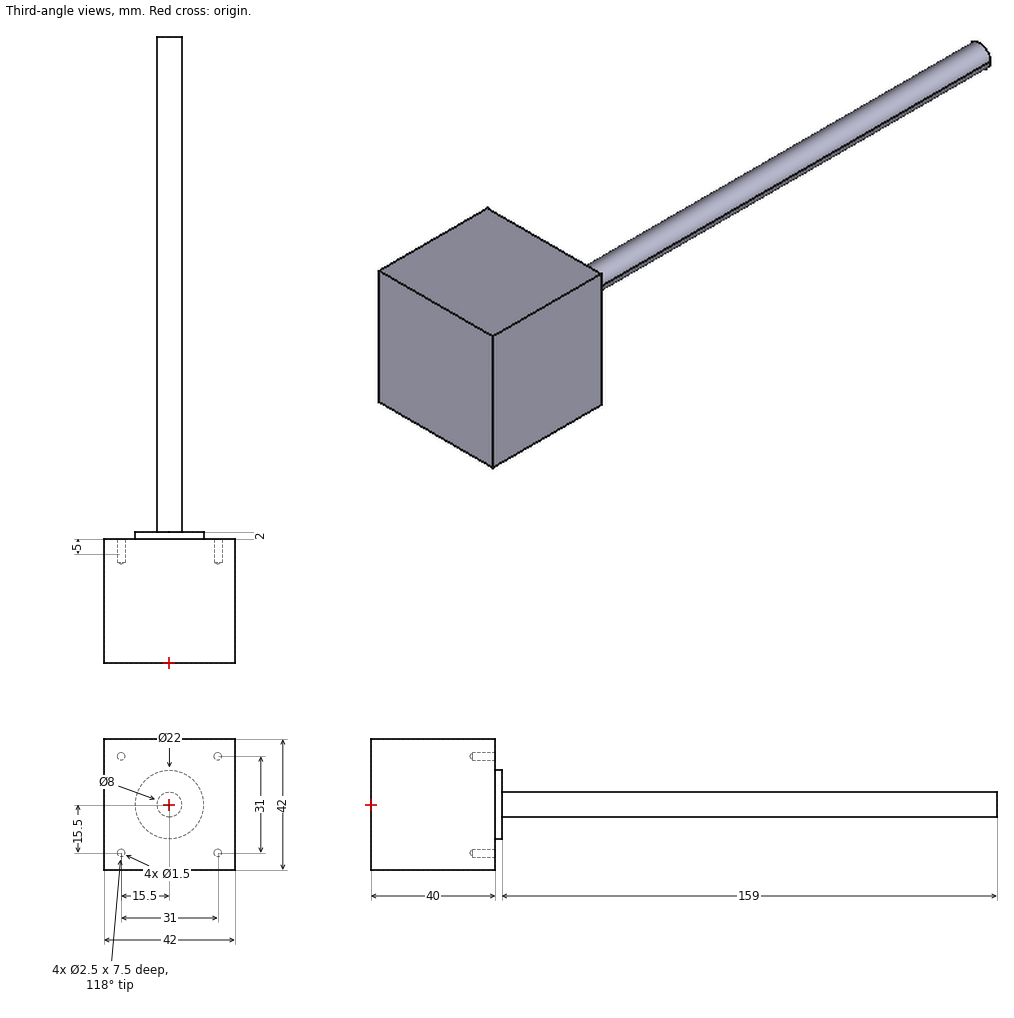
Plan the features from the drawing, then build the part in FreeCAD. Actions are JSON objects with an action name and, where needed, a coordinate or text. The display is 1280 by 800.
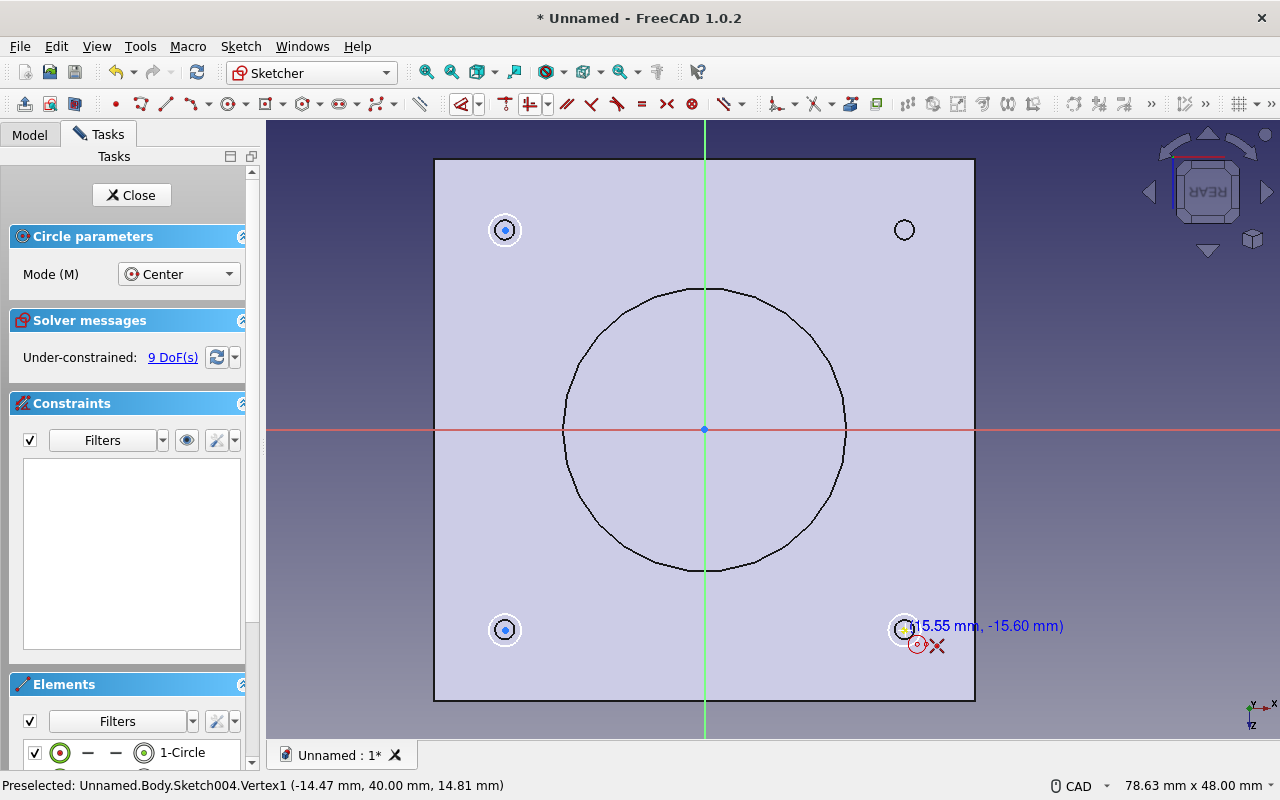
{"action": "scroll", "coordinate": [905, 230], "scroll_direction": "up", "scroll_amount": 2}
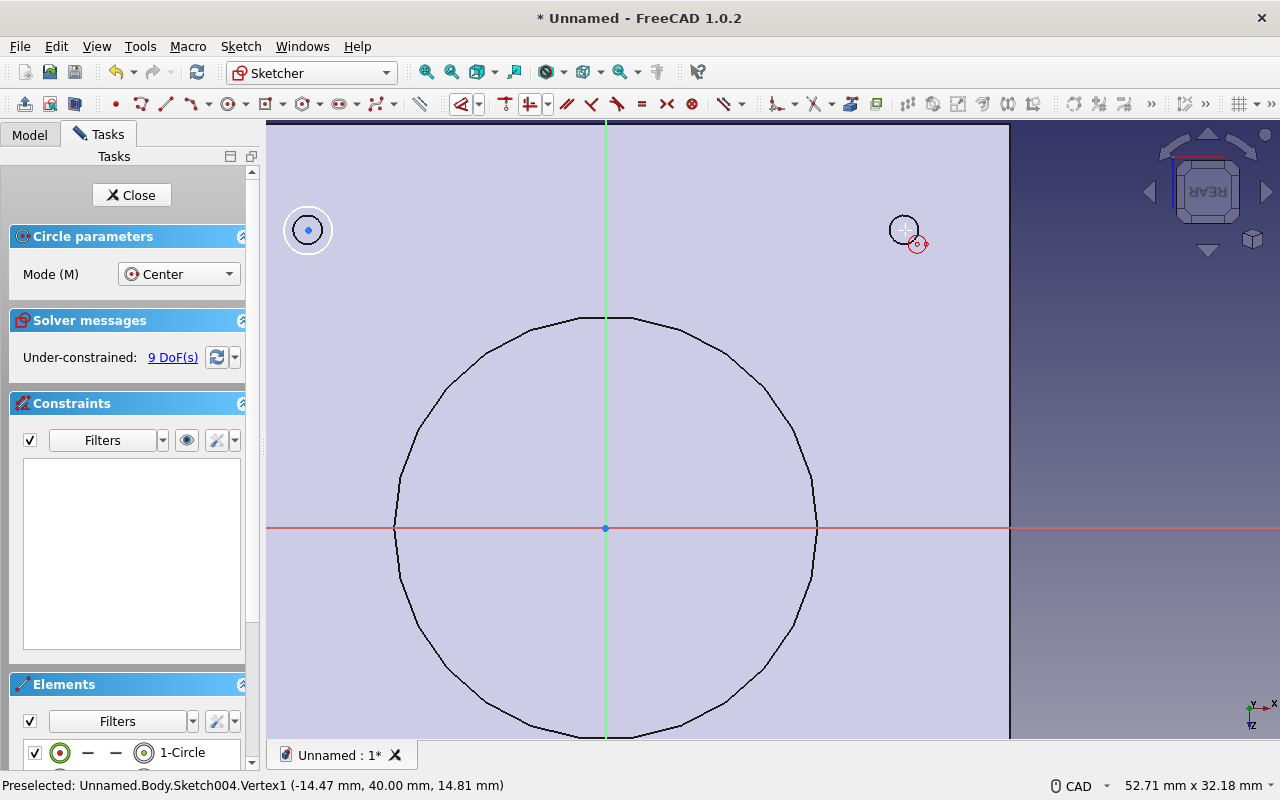
{"action": "left_click", "coordinate": [904, 230]}
{"action": "left_click", "coordinate": [921, 213]}
{"action": "key", "text": "Escape"}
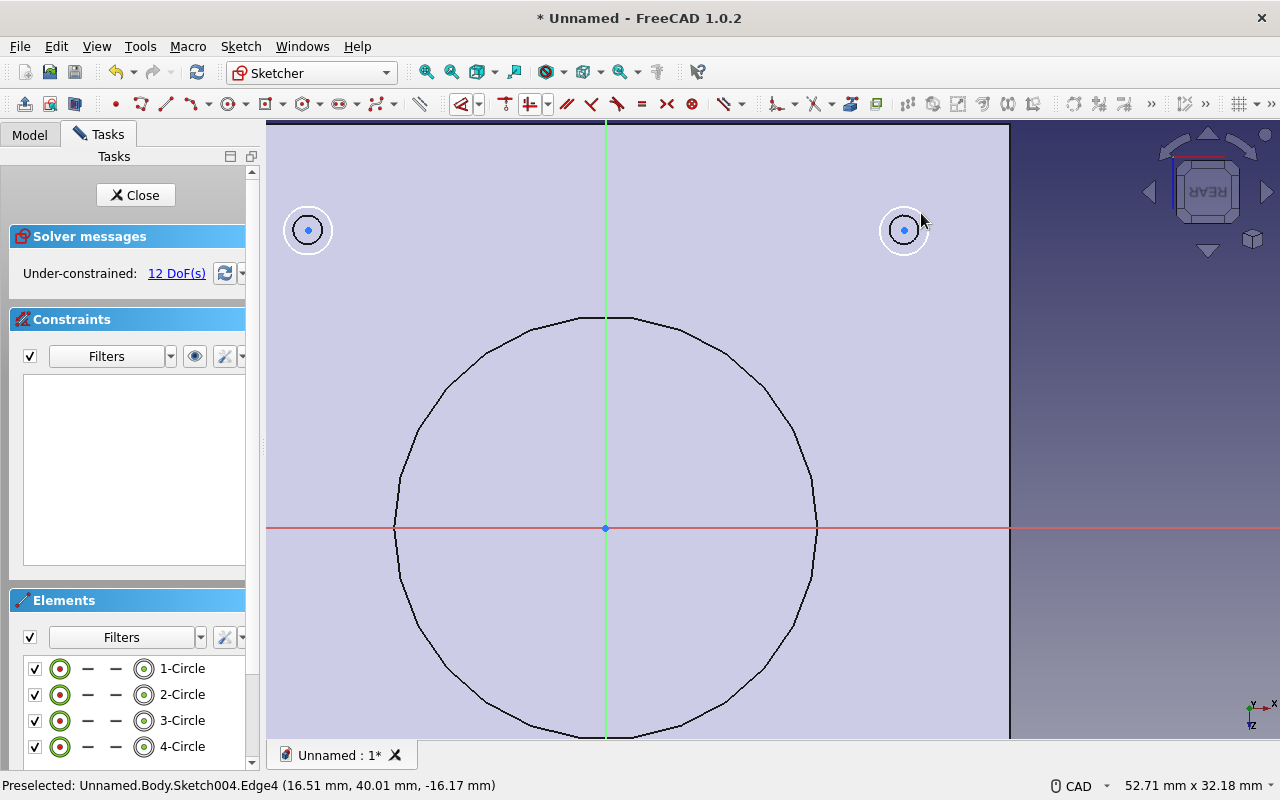
{"action": "left_click", "coordinate": [325, 213]}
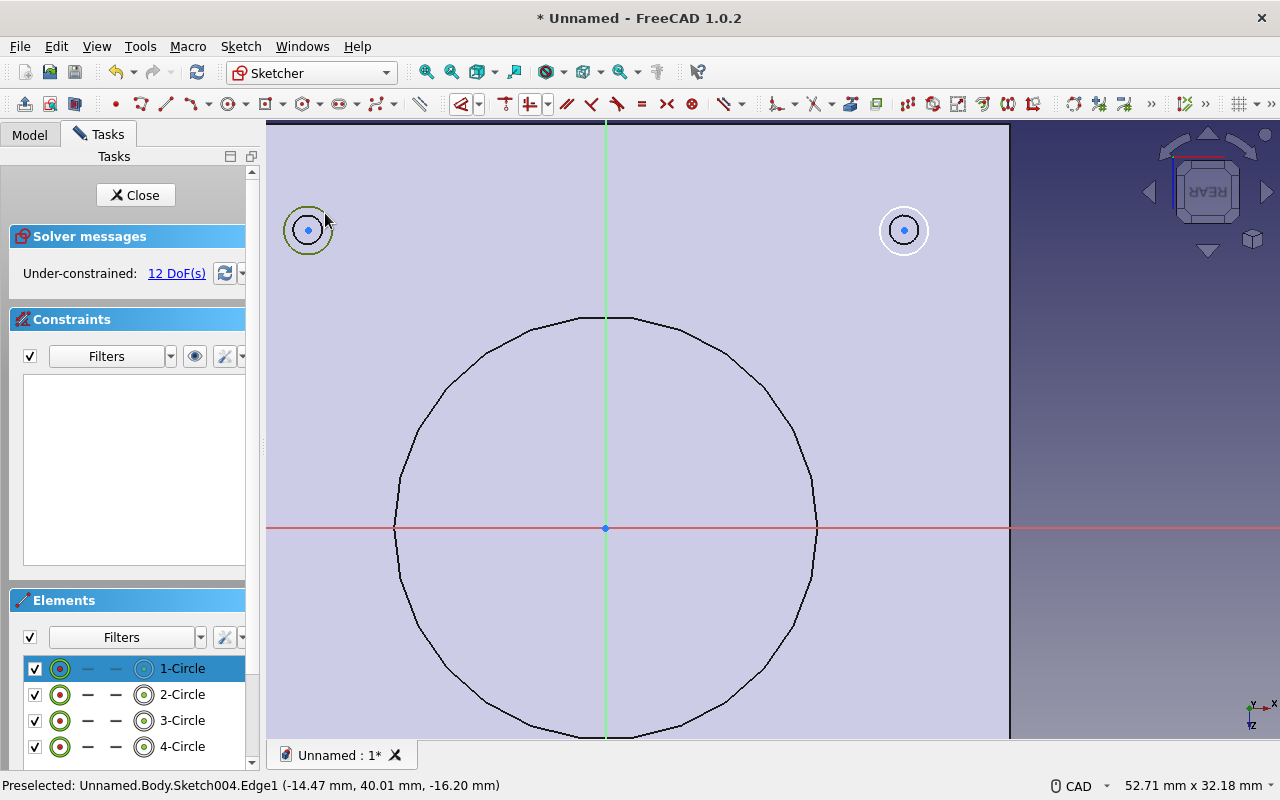
{"action": "scroll", "coordinate": [905, 229], "scroll_direction": "down", "scroll_amount": 2}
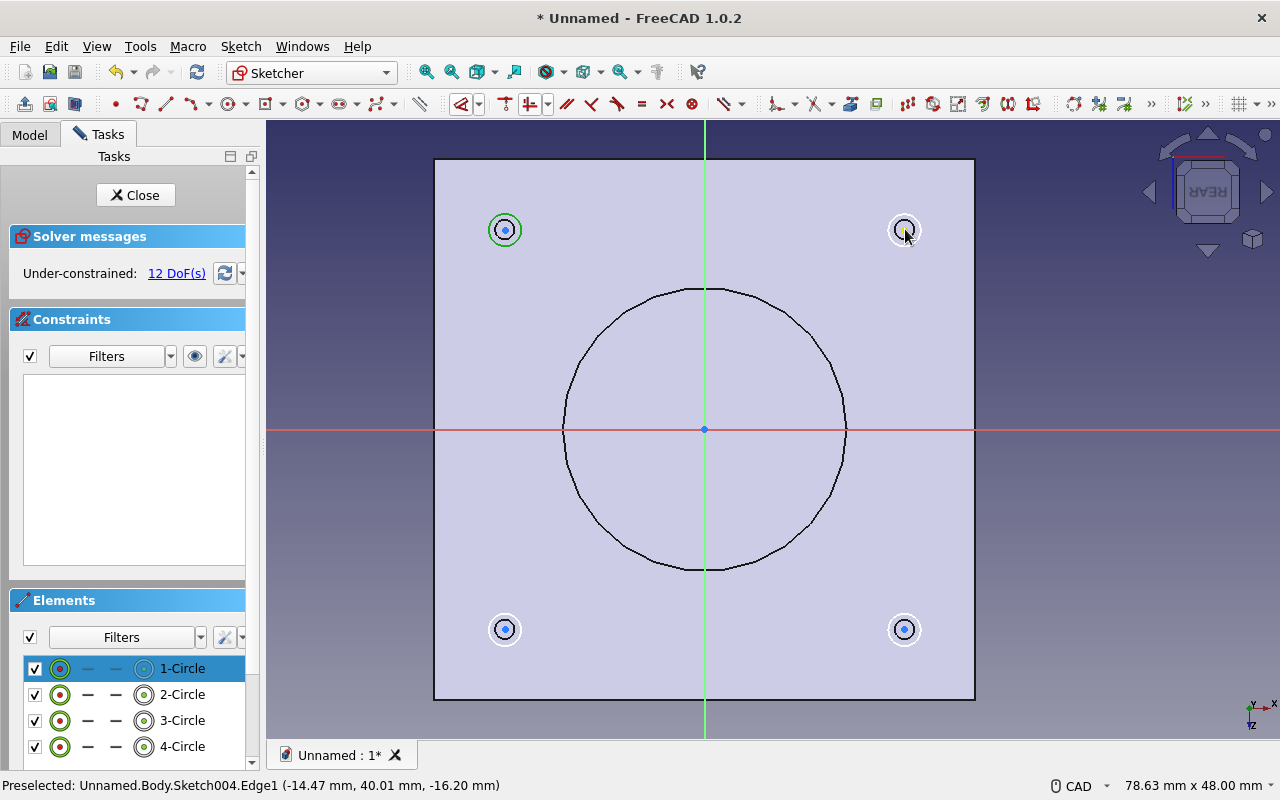
{"action": "left_click", "coordinate": [916, 619]}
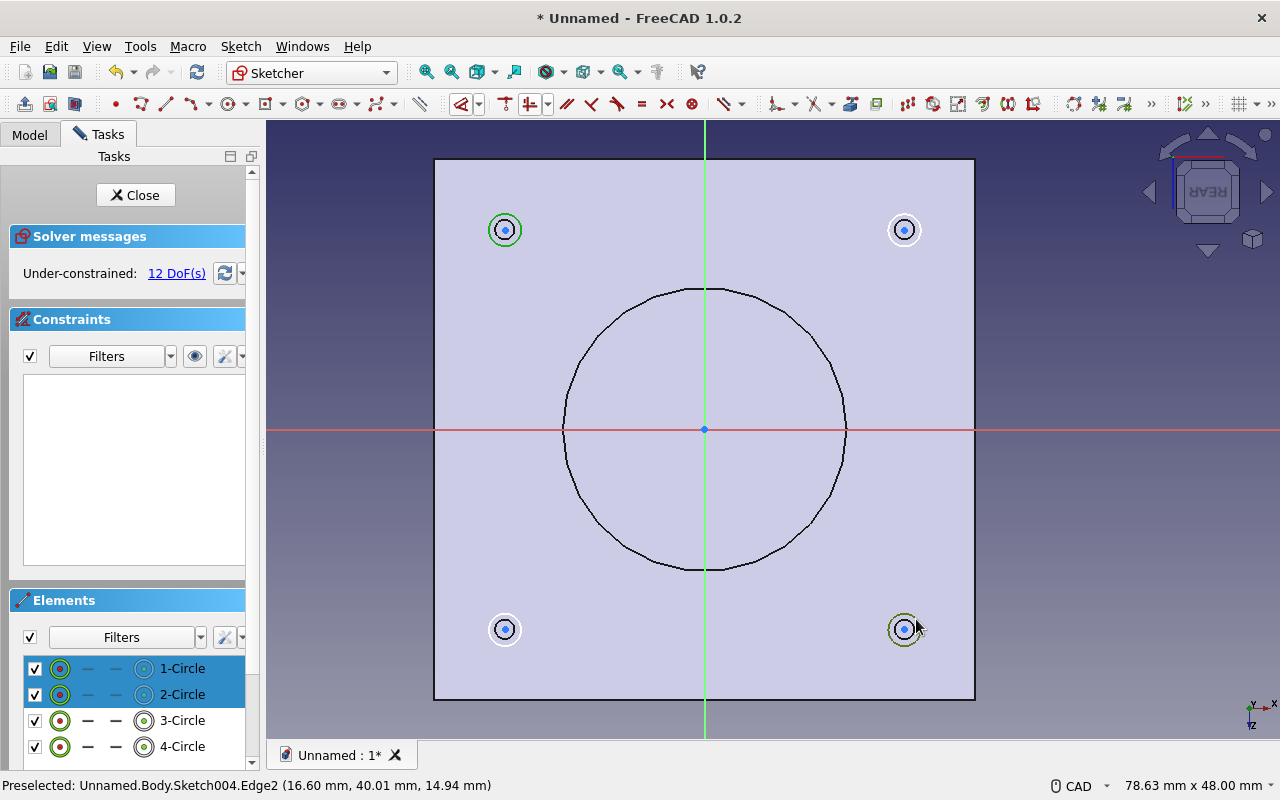
{"action": "left_click", "coordinate": [516, 619]}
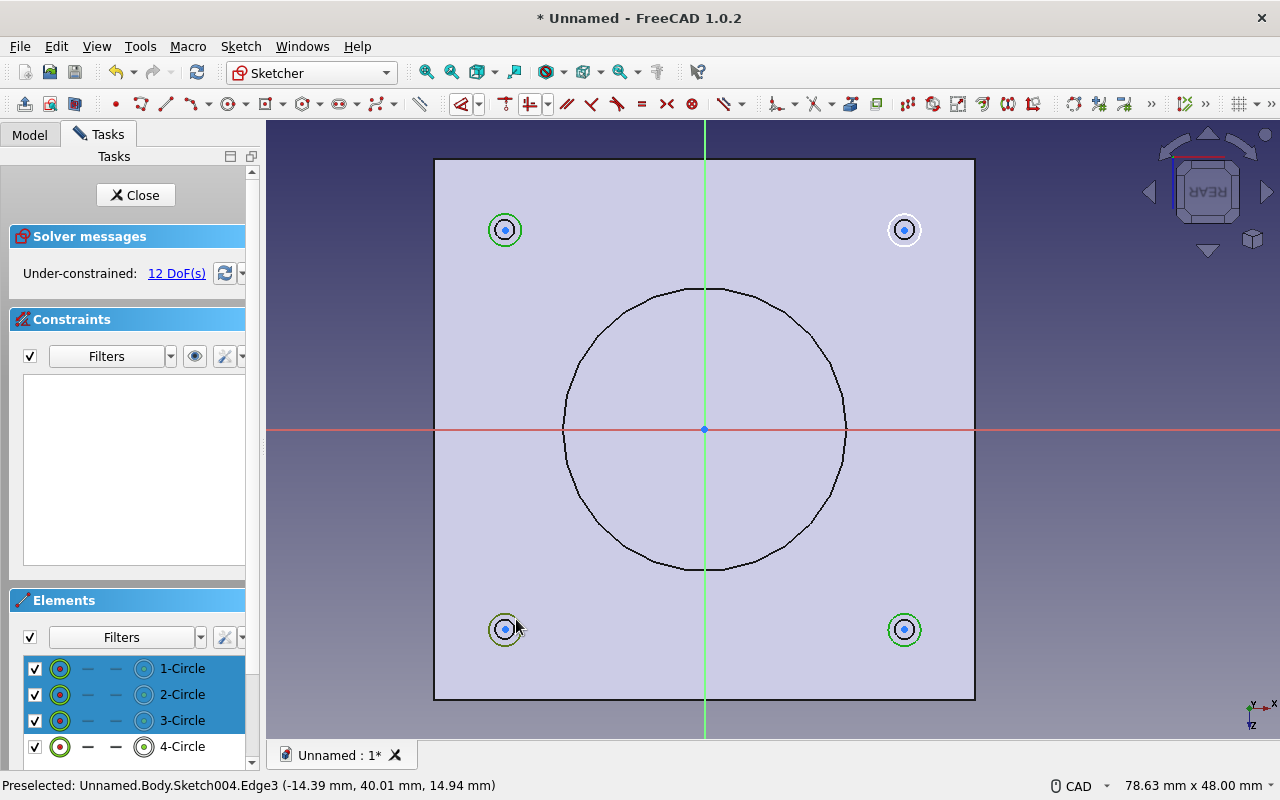
{"action": "left_click", "coordinate": [916, 219]}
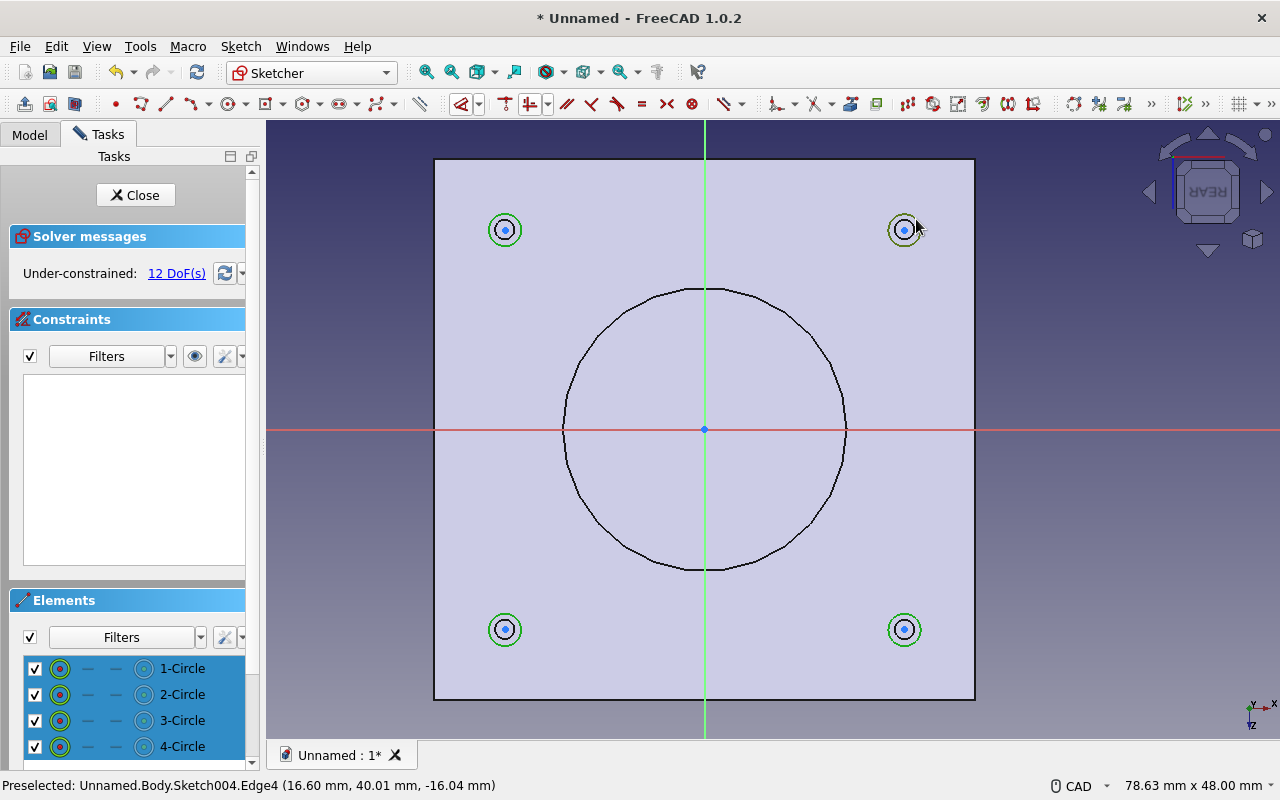
{"action": "key", "text": "e"}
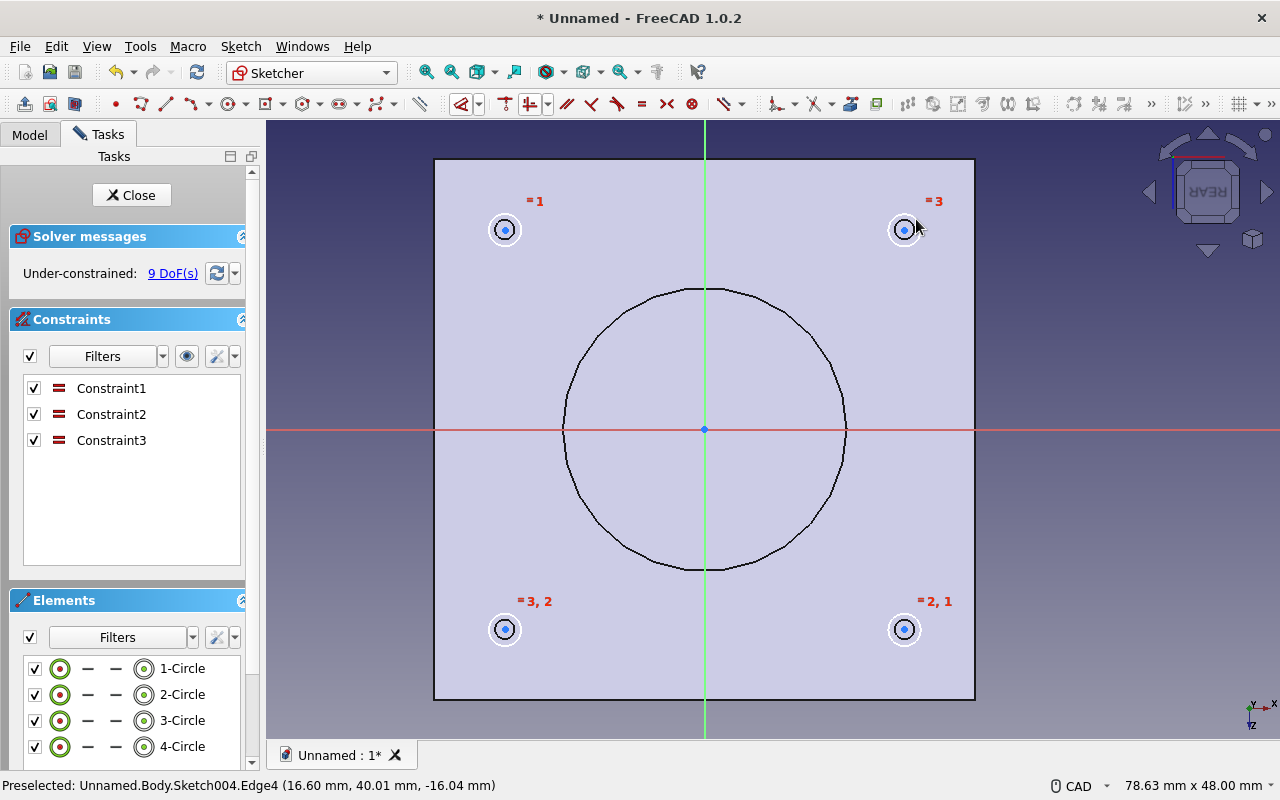
{"action": "left_click", "coordinate": [505, 230]}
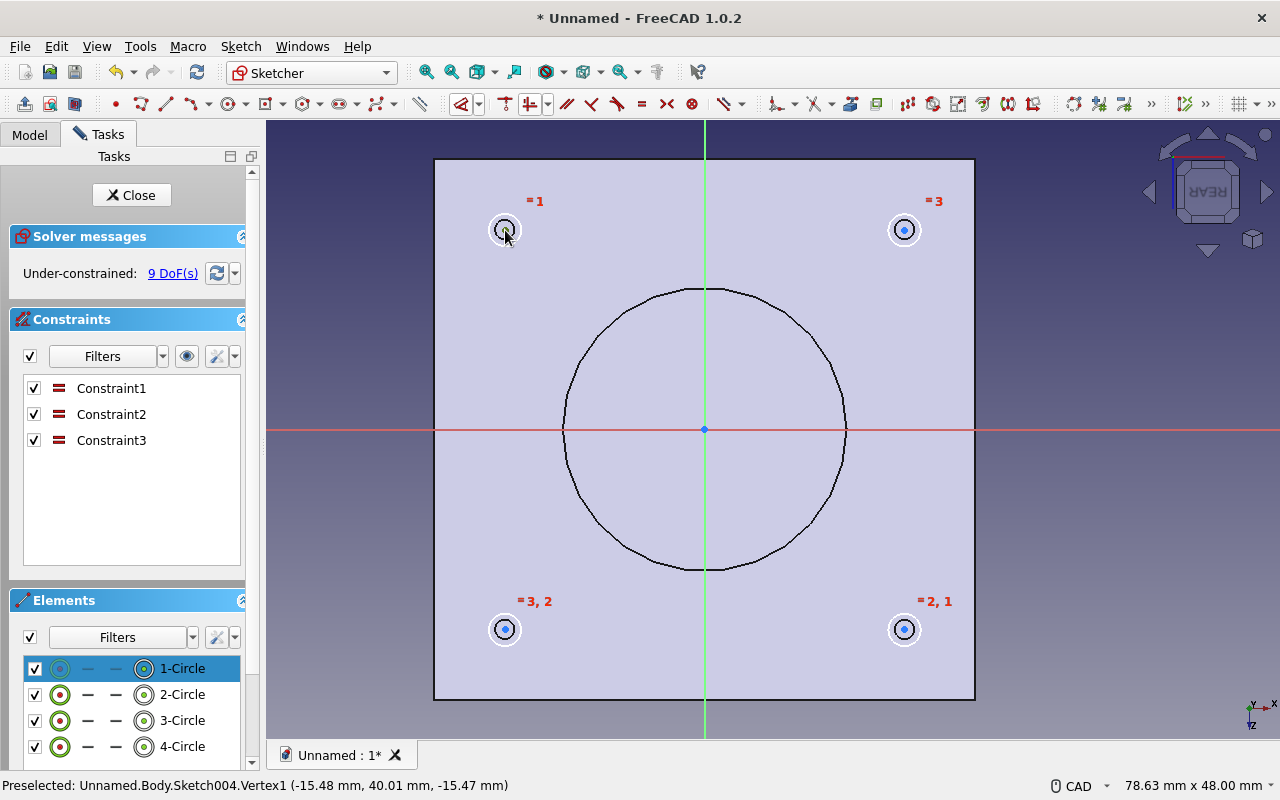
{"action": "left_click", "coordinate": [505, 630]}